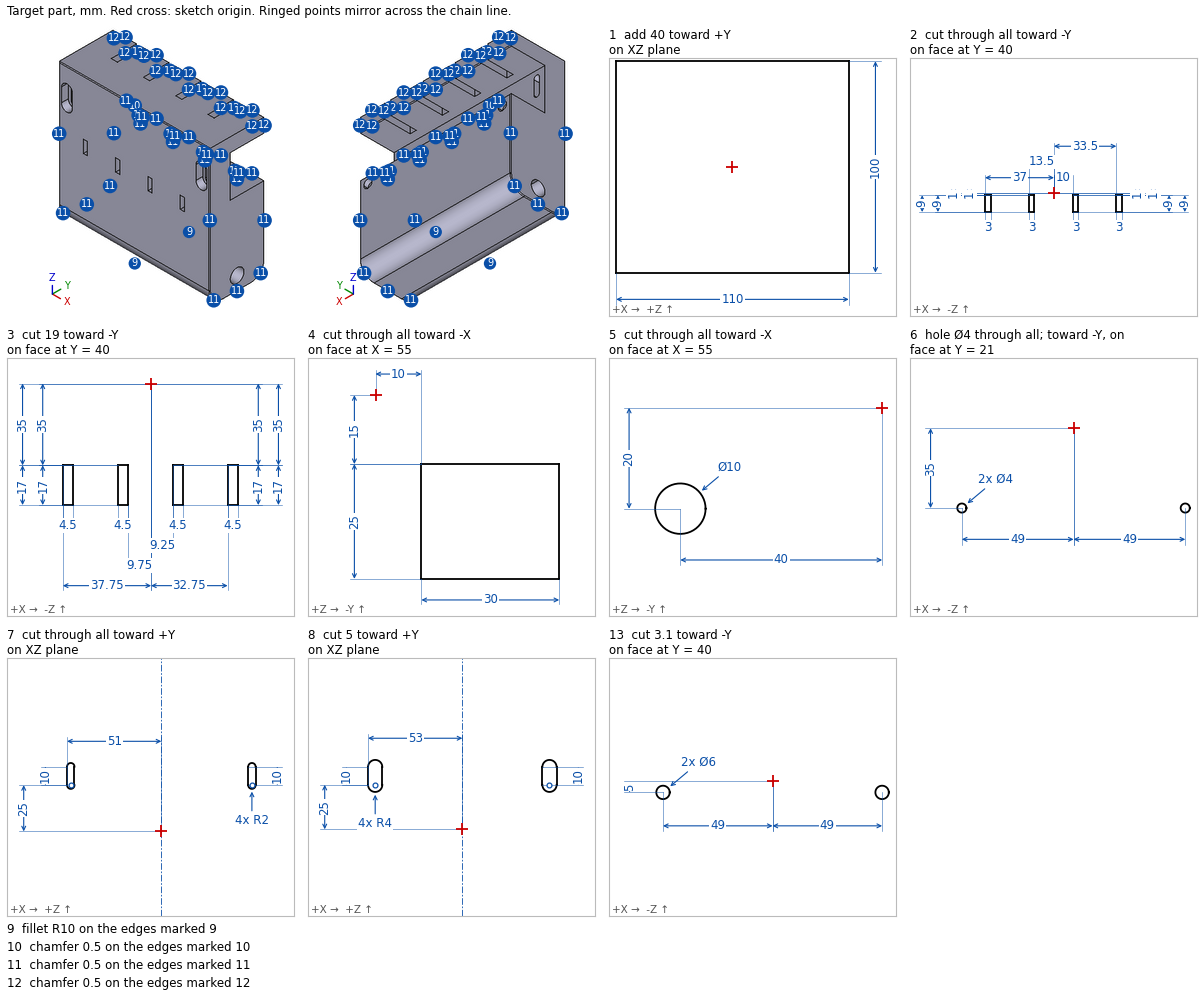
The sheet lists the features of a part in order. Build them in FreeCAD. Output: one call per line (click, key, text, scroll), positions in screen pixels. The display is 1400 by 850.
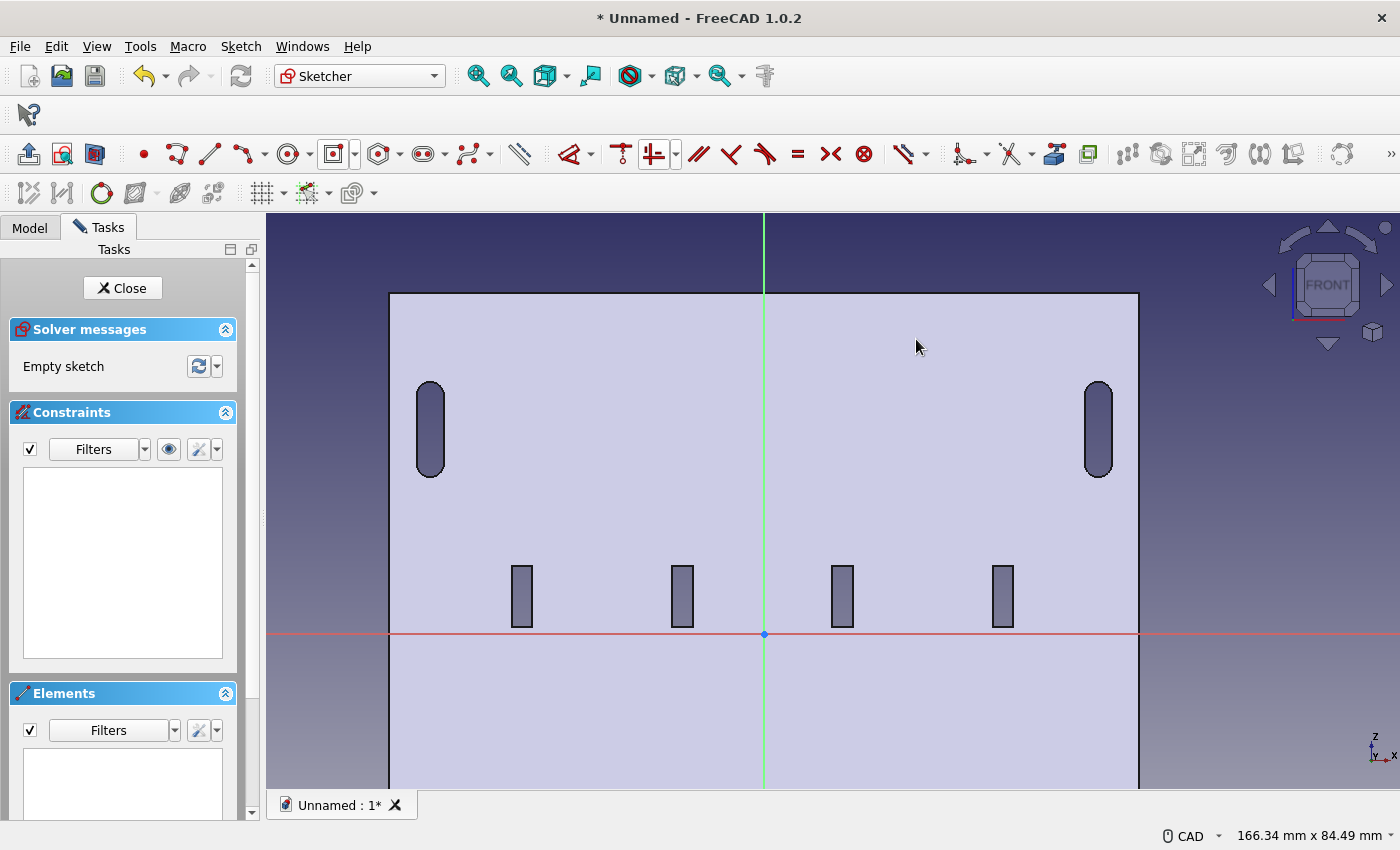
click(430, 464)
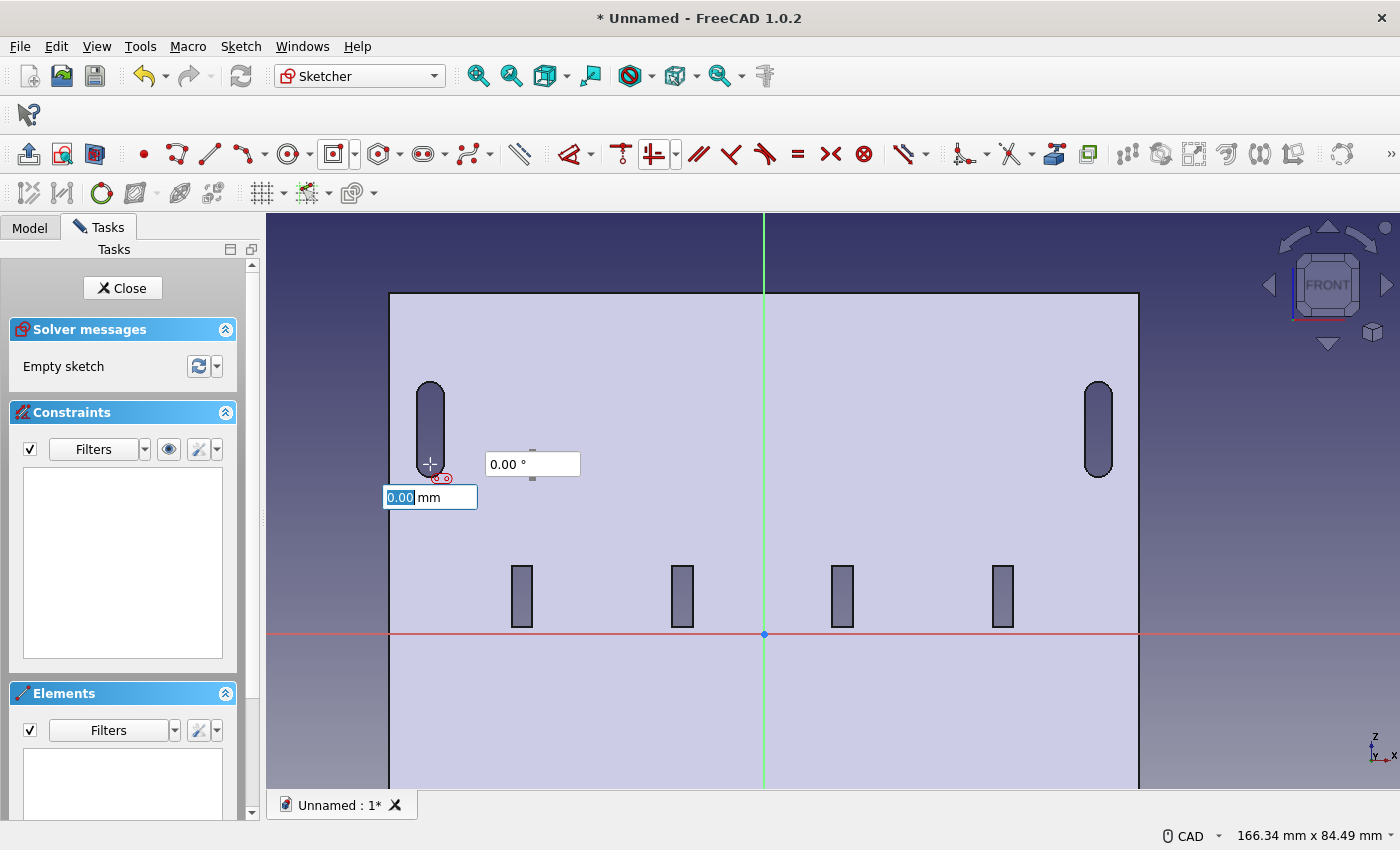
click(430, 395)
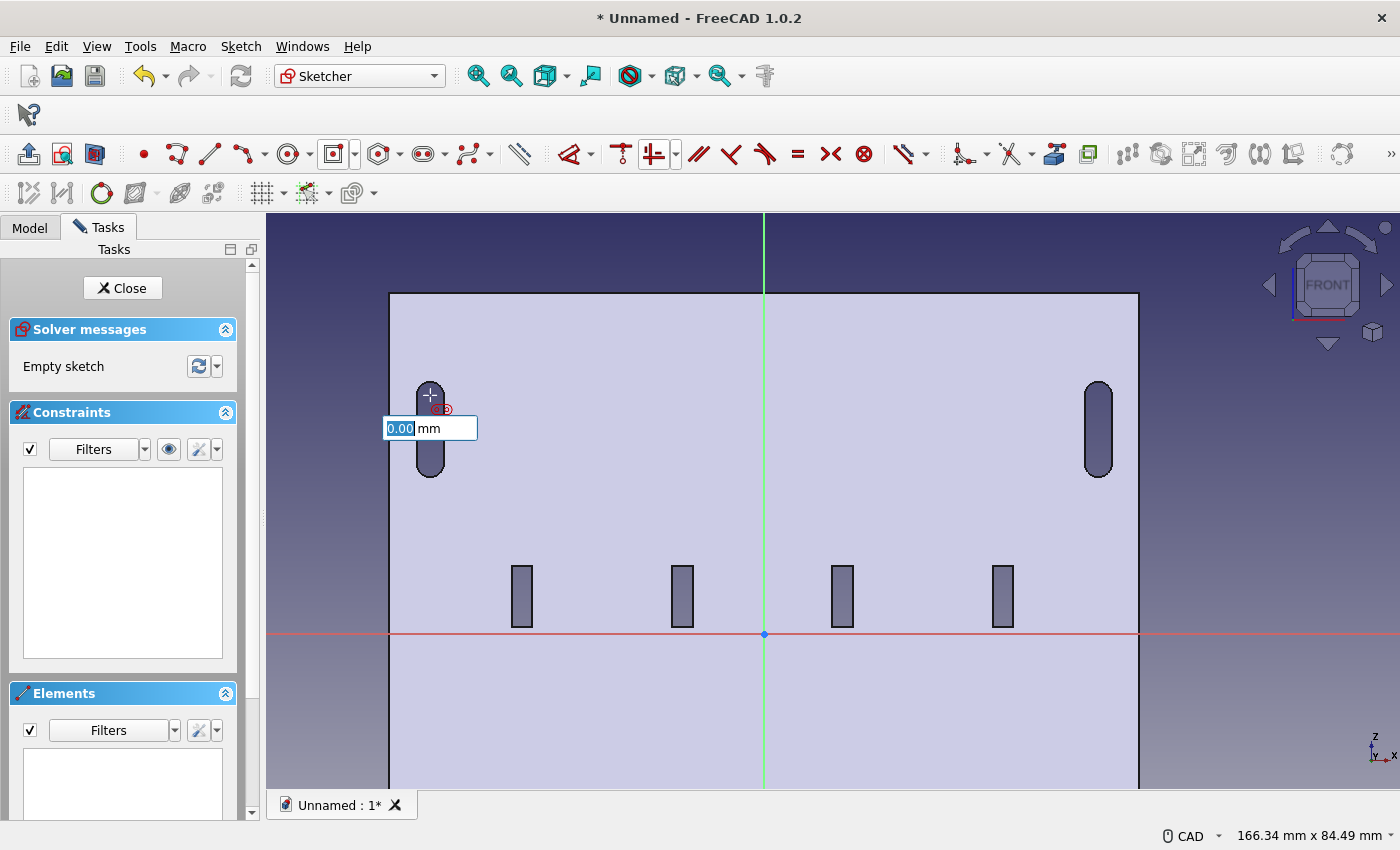
click(403, 429)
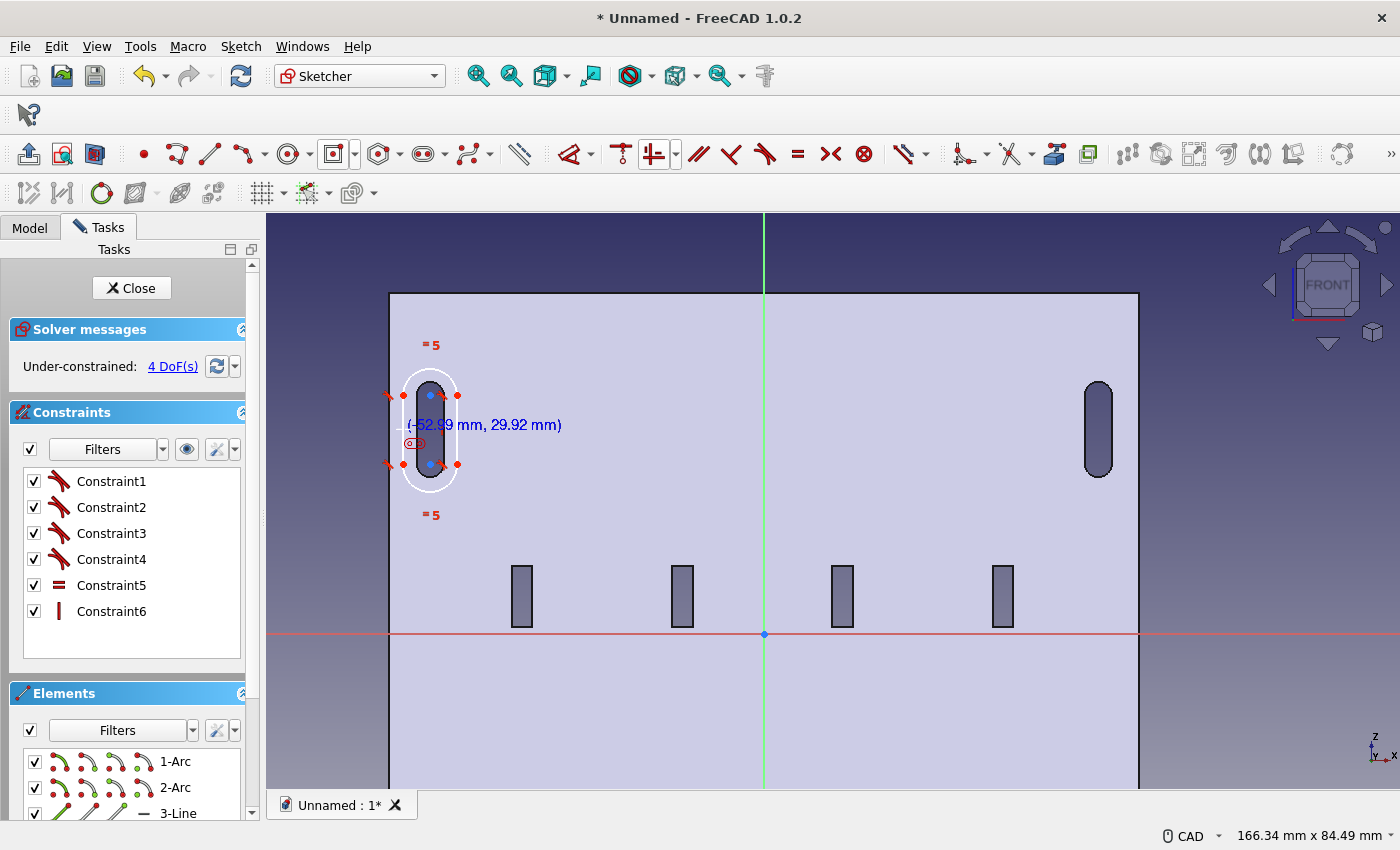
click(1098, 464)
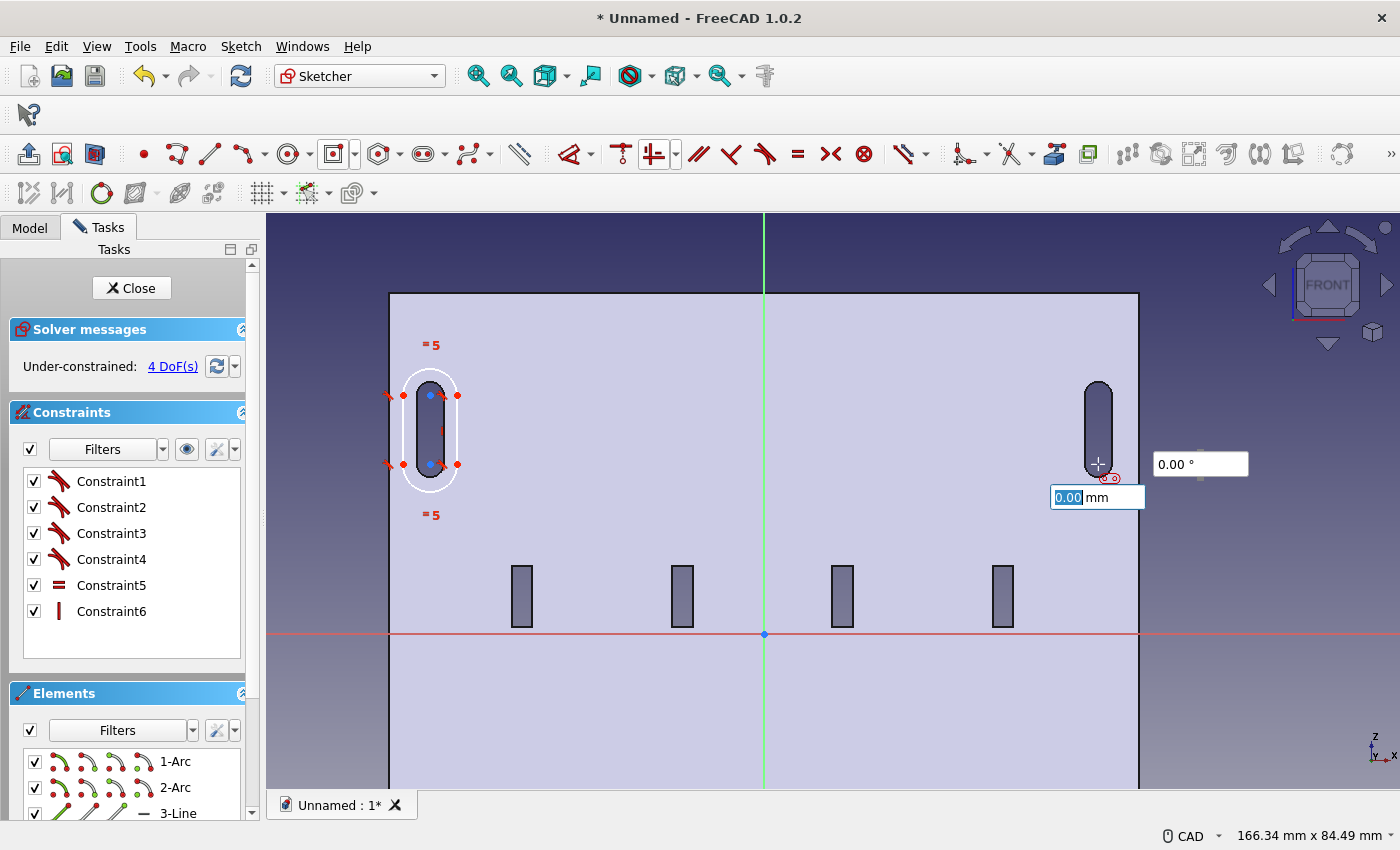
click(1098, 395)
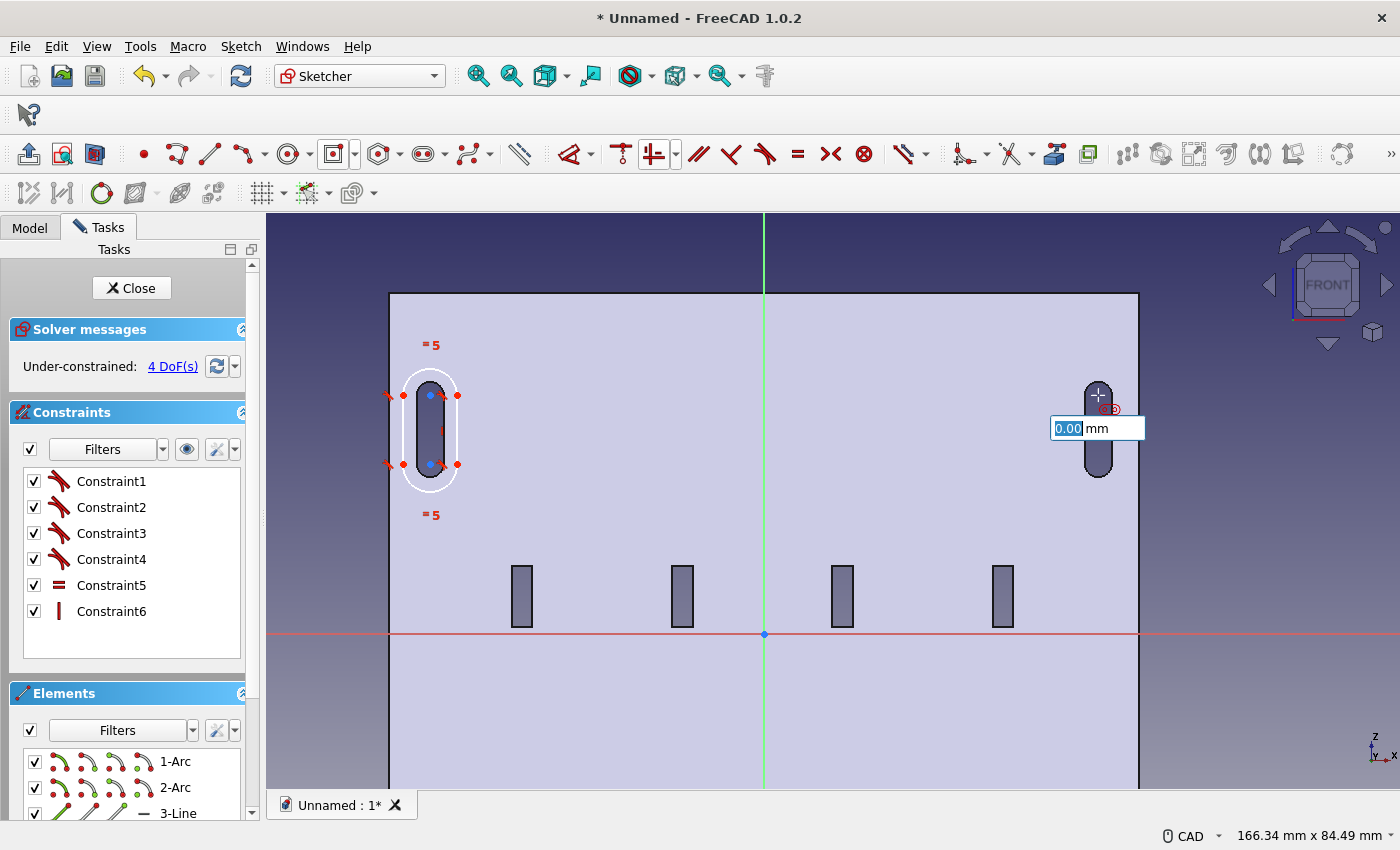
click(1071, 429)
key(Escape)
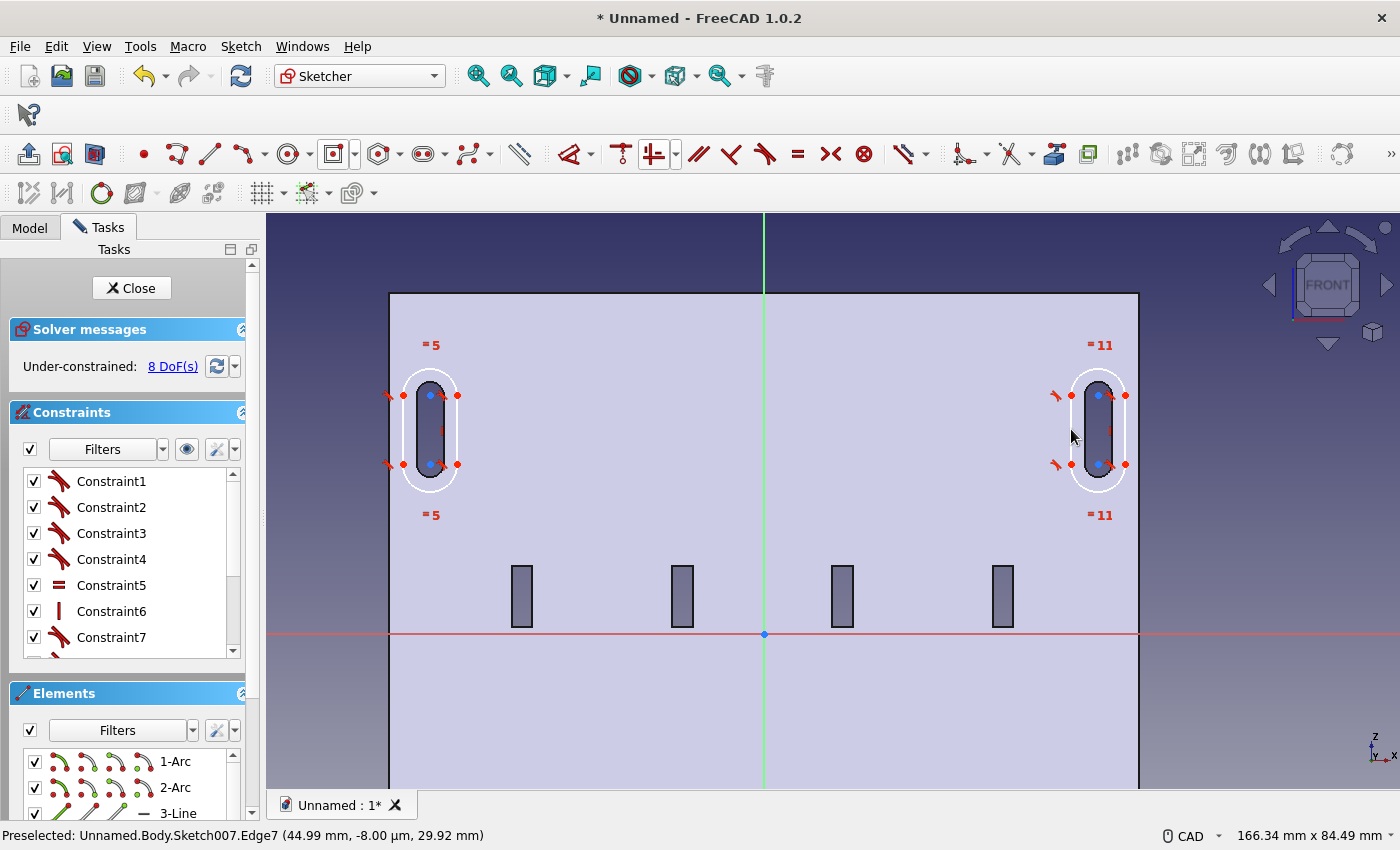
click(414, 487)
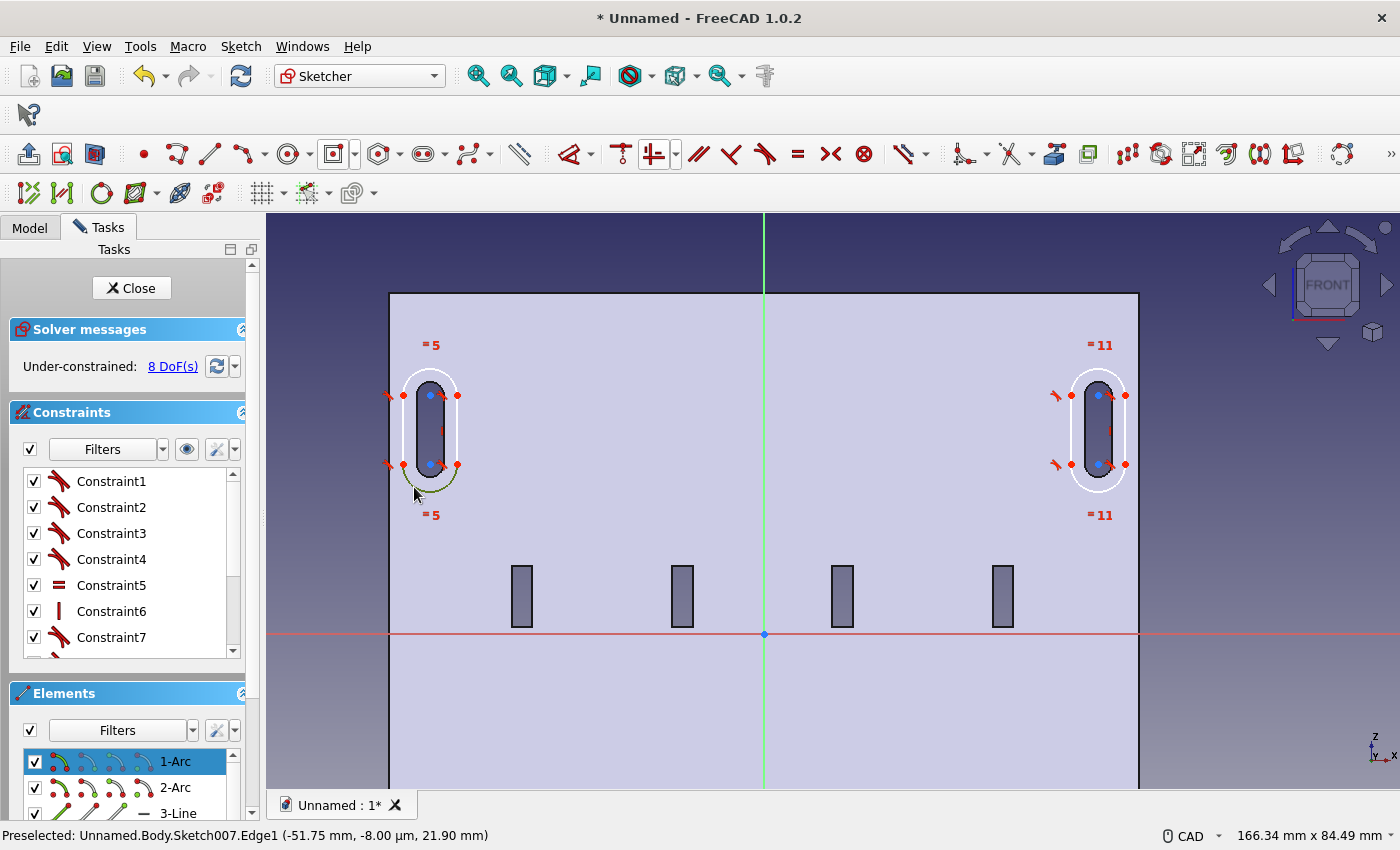
click(1082, 487)